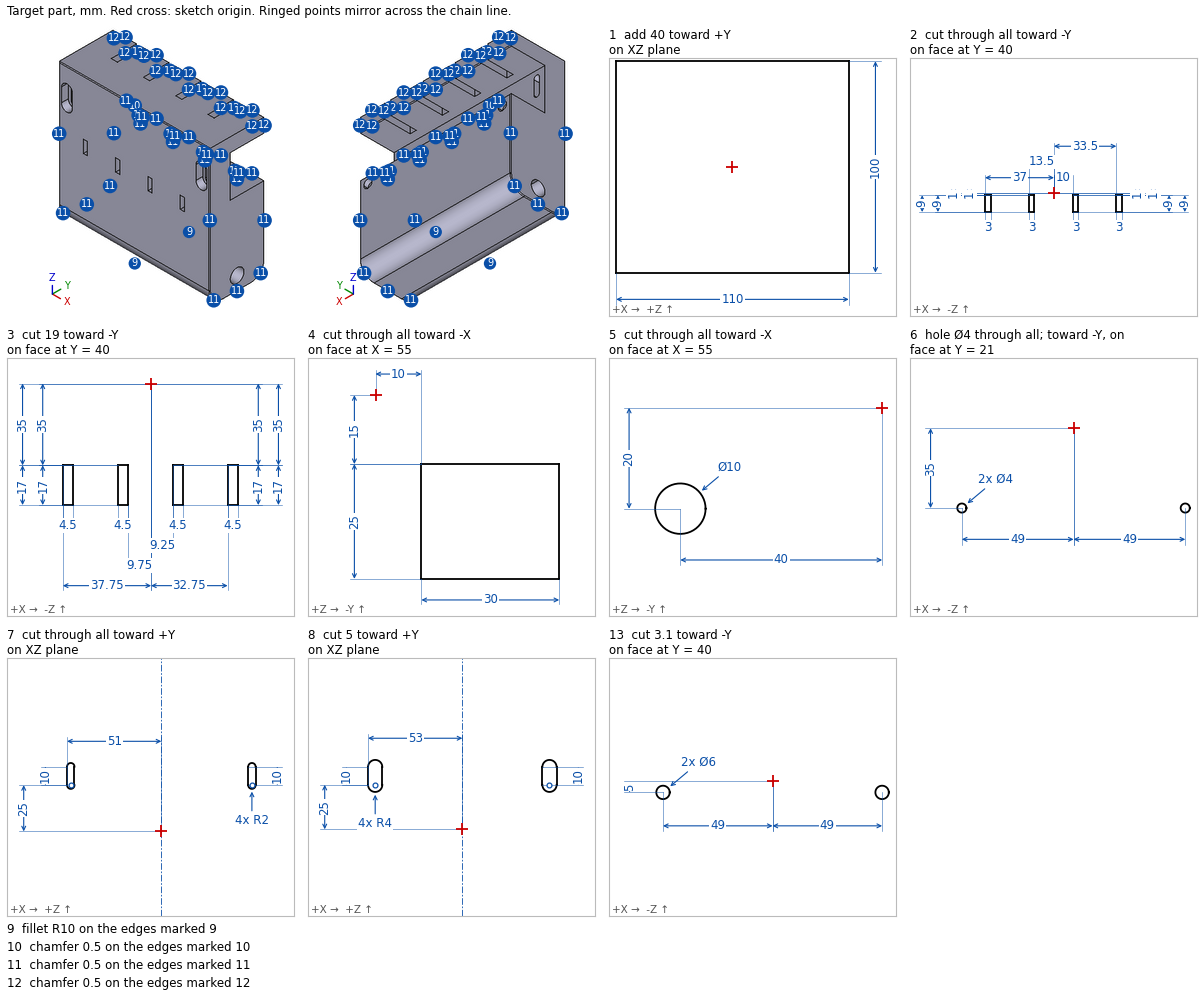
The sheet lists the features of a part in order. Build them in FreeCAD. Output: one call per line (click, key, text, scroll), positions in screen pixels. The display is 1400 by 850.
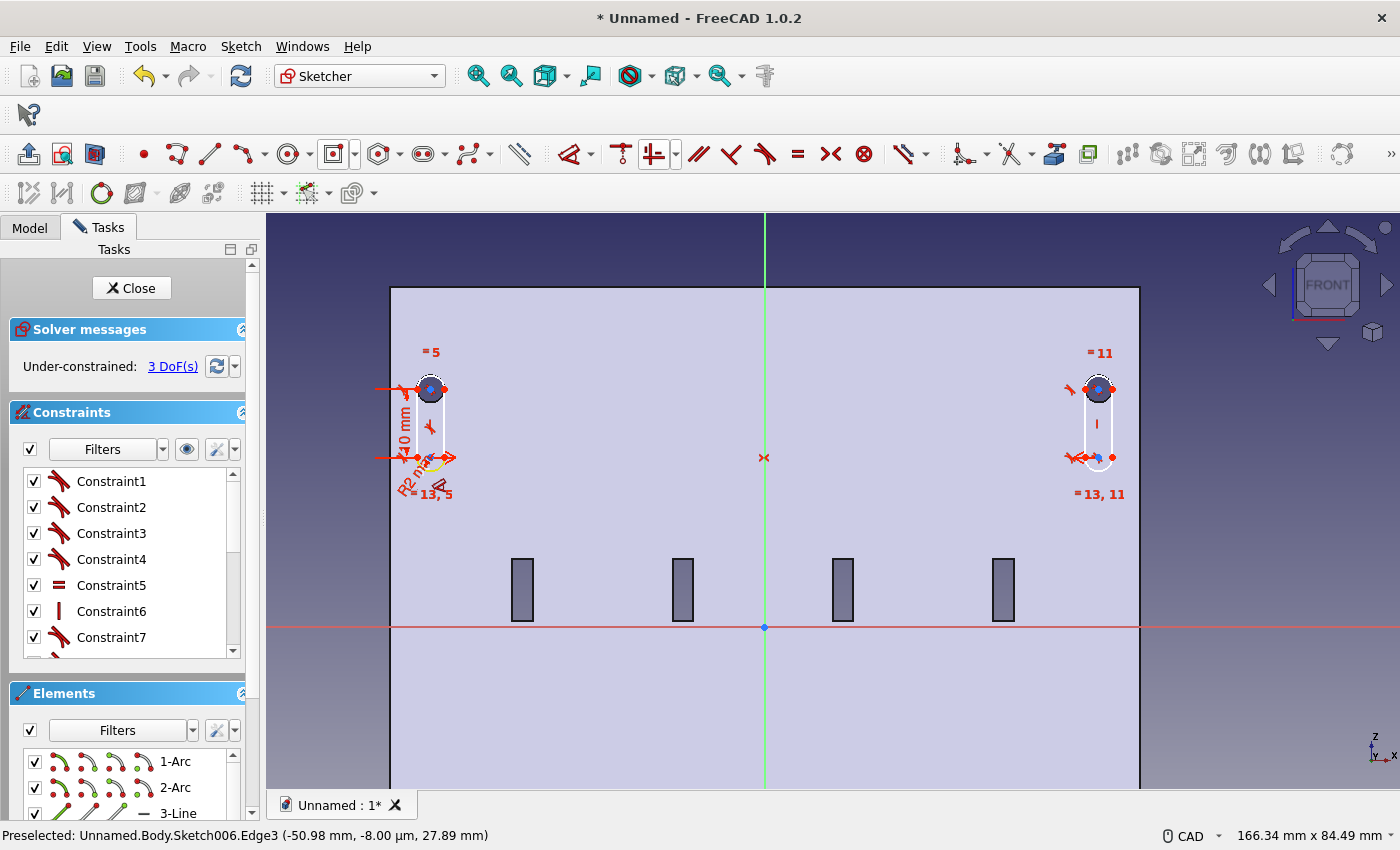
click(1085, 437)
click(1051, 424)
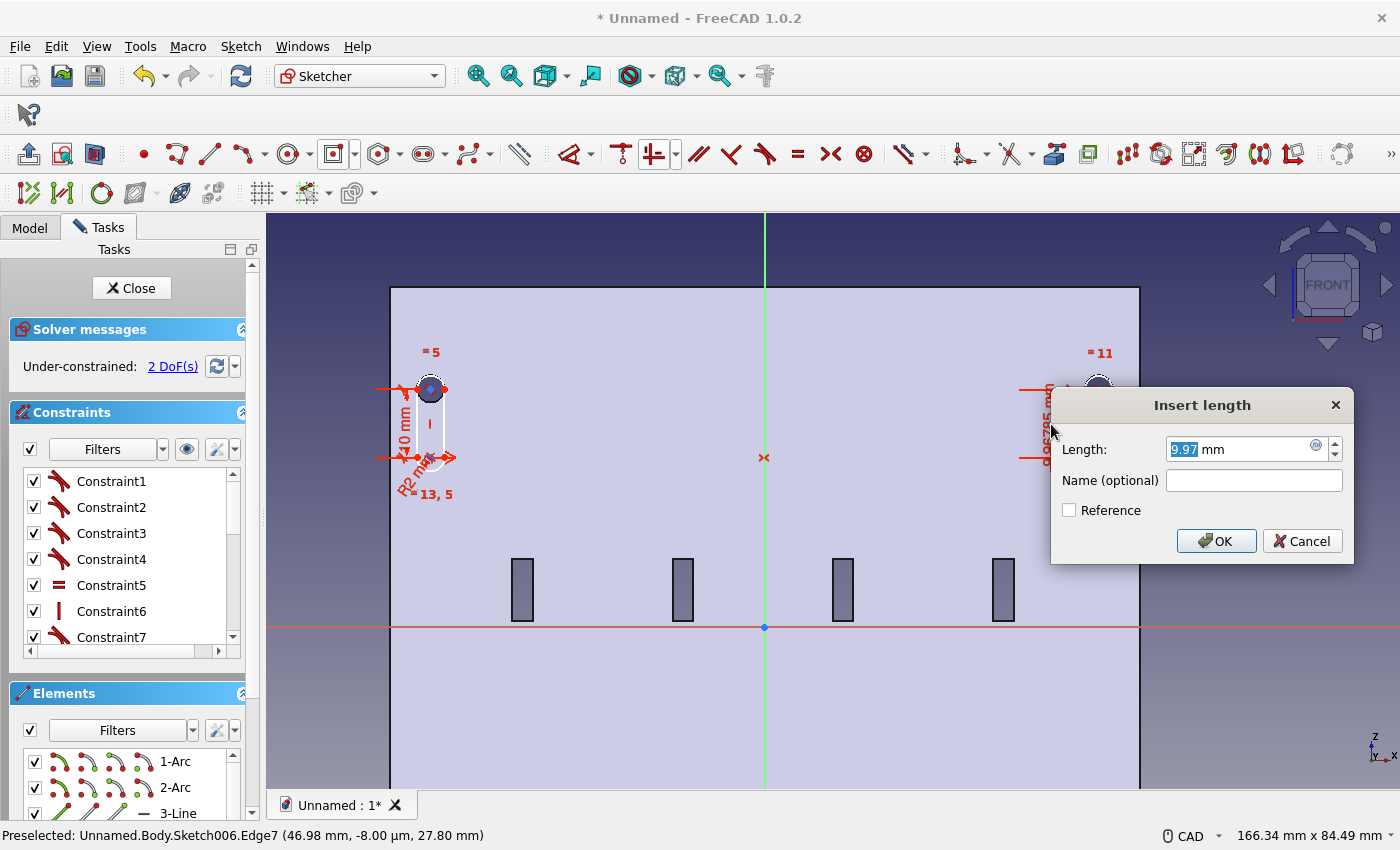
text(10)
key(Return)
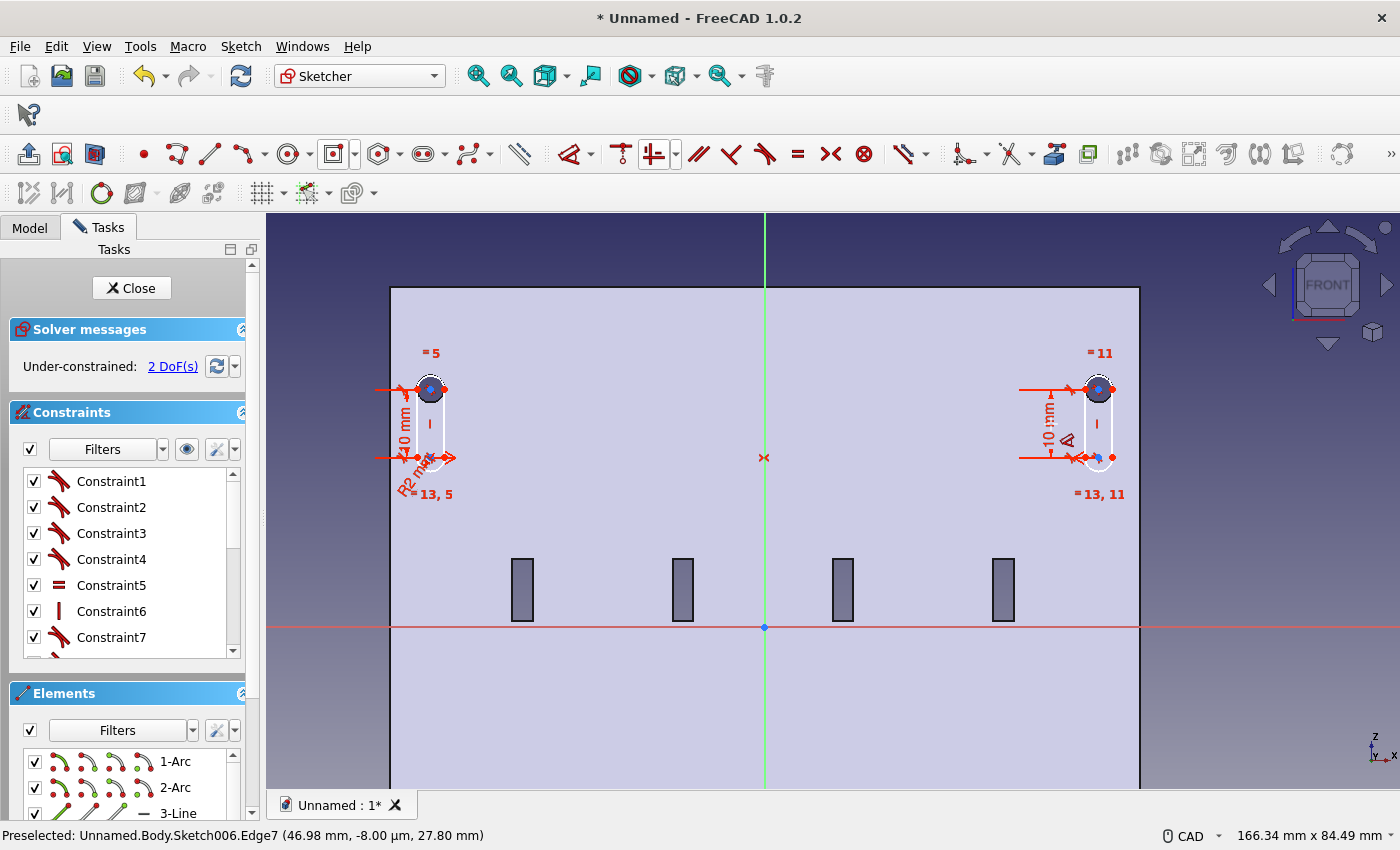
click(417, 458)
click(591, 661)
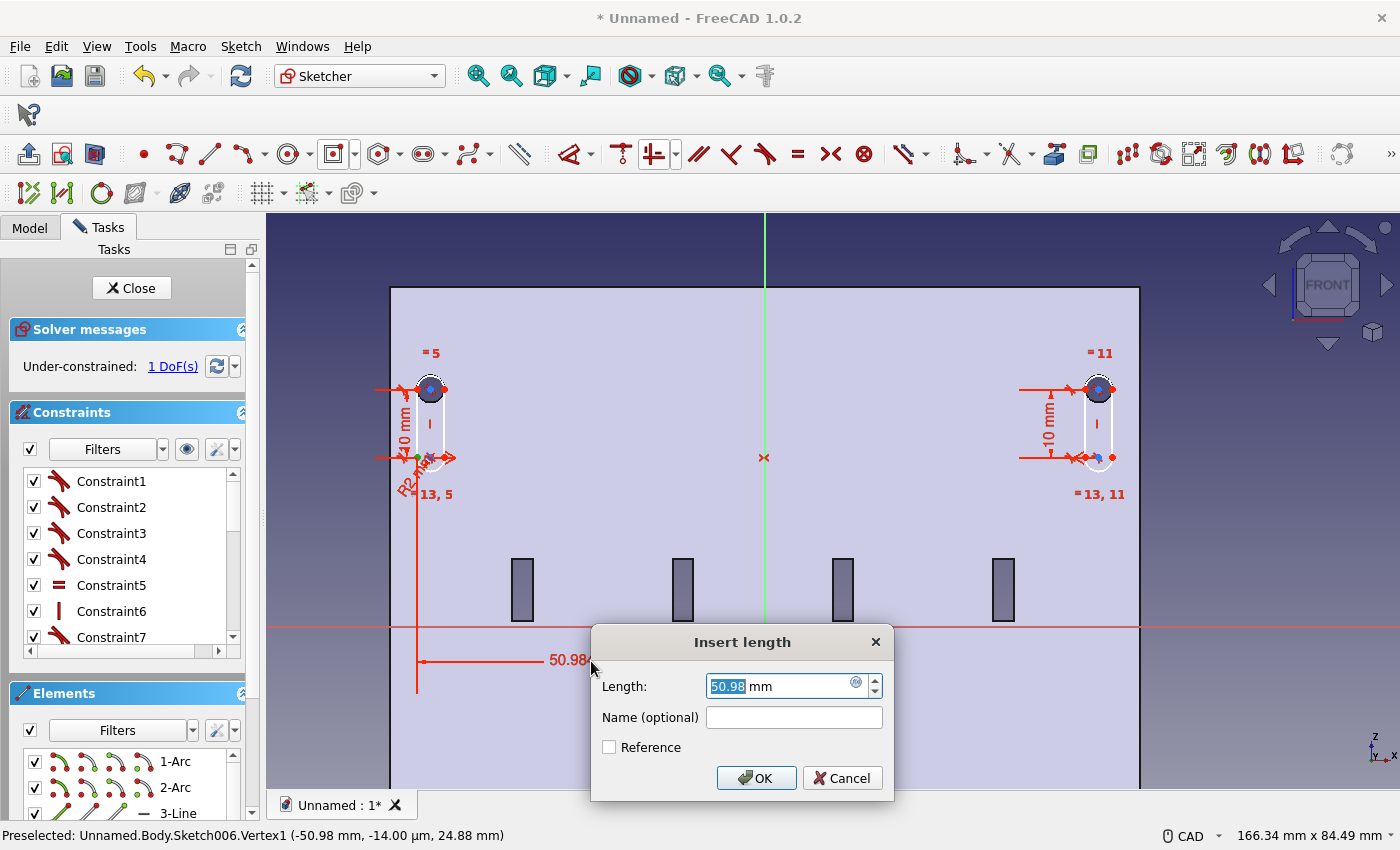
text(51)
key(Return)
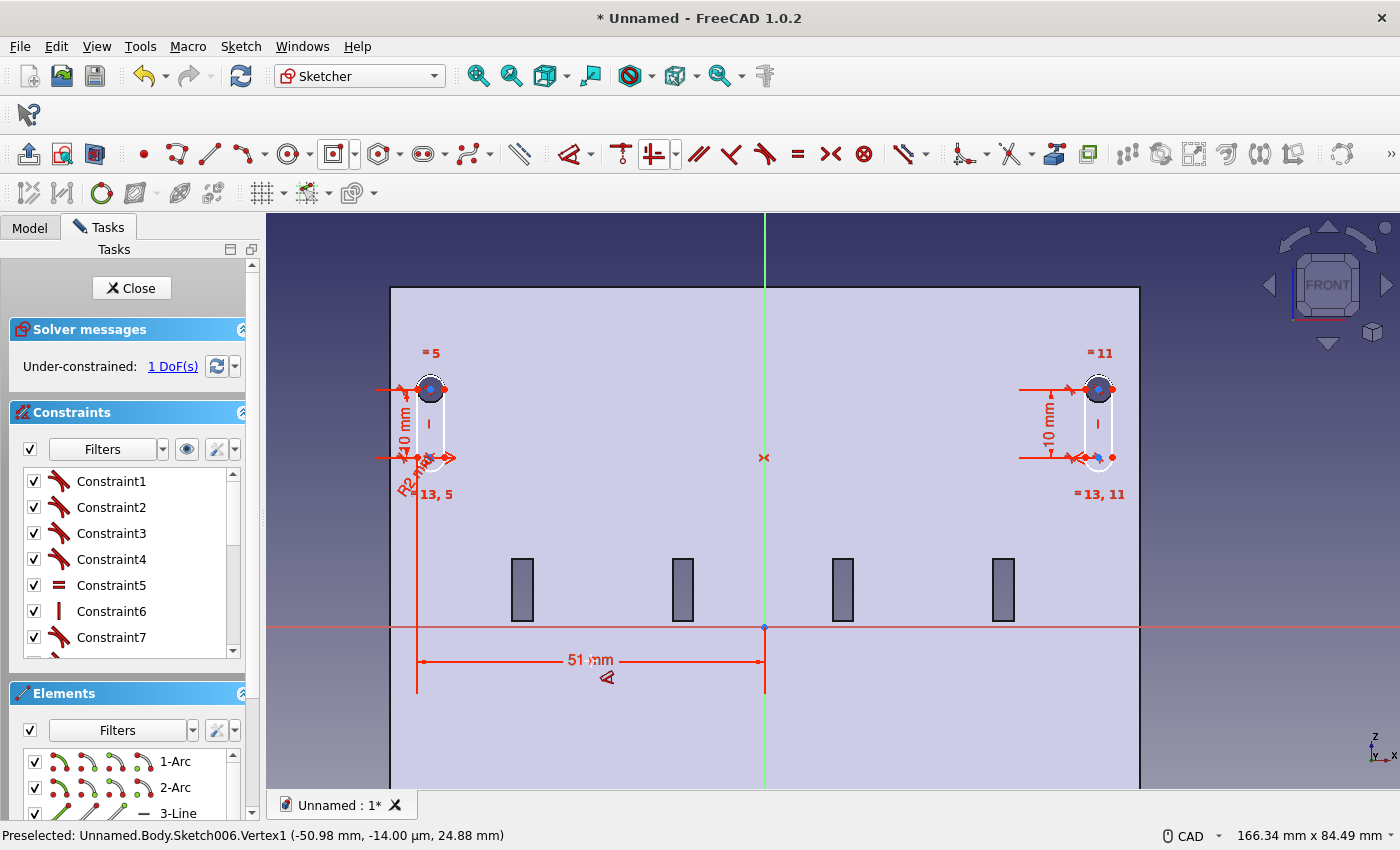
click(417, 458)
click(383, 543)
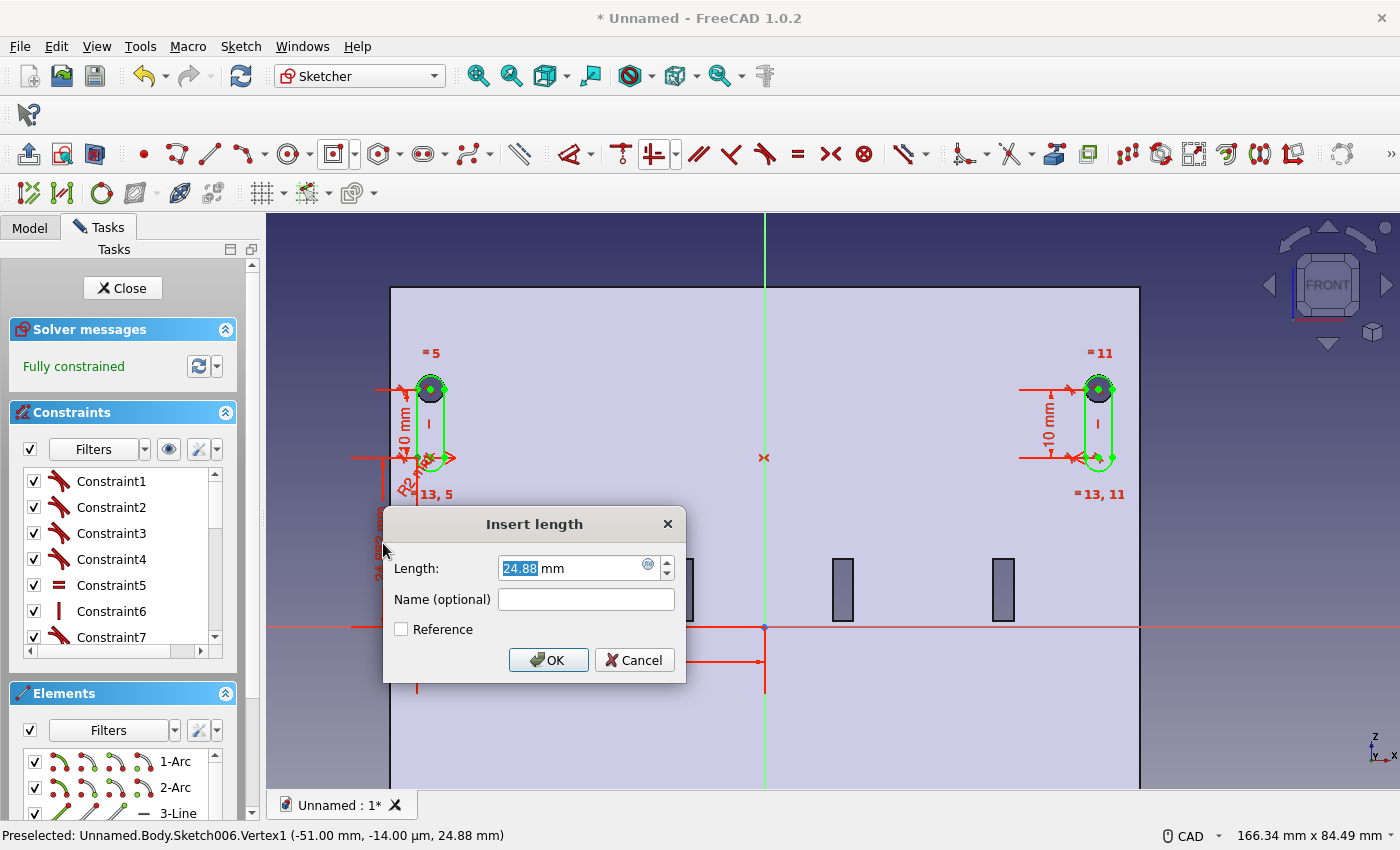
text(25)
key(Return)
key(Escape)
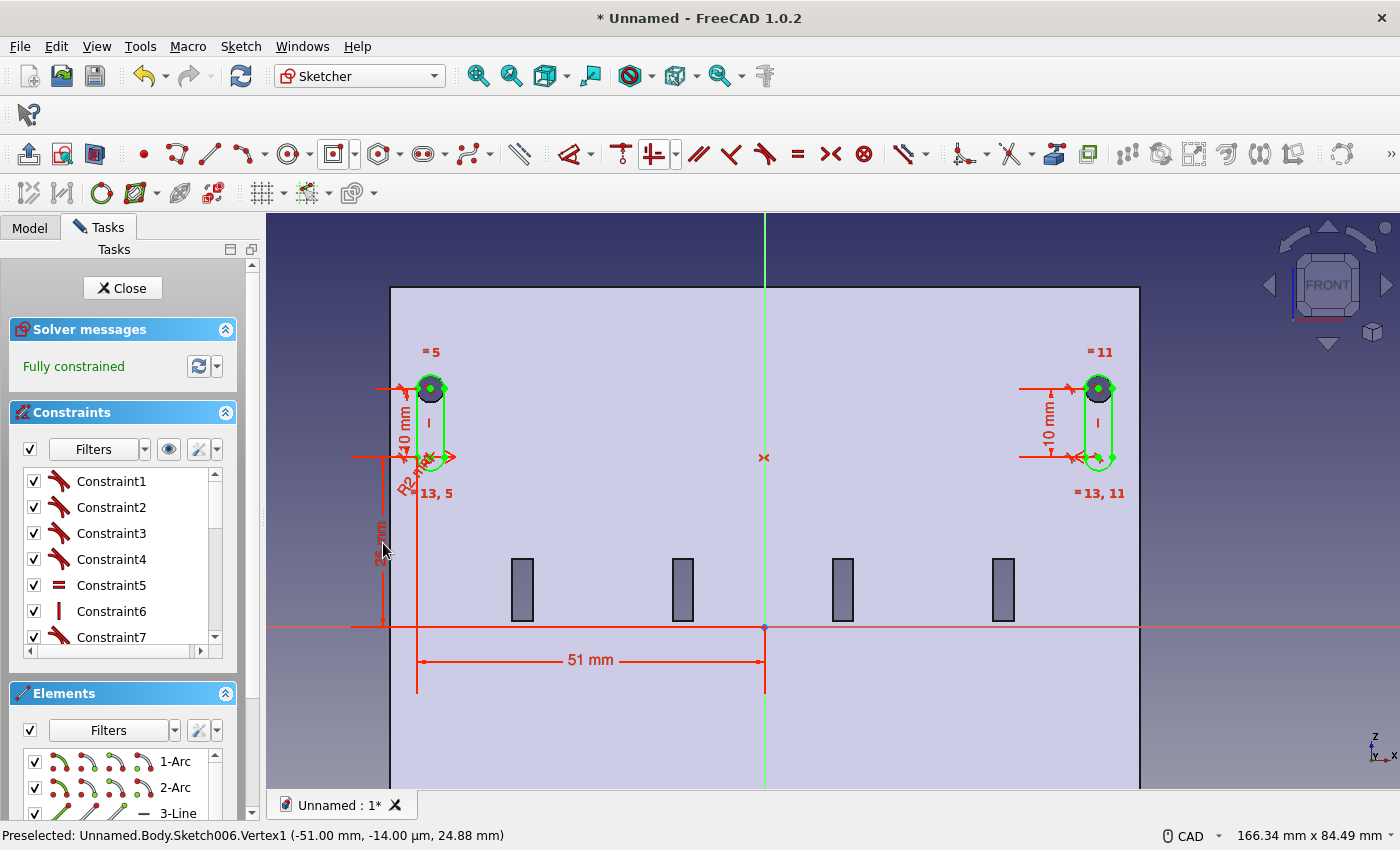
click(123, 288)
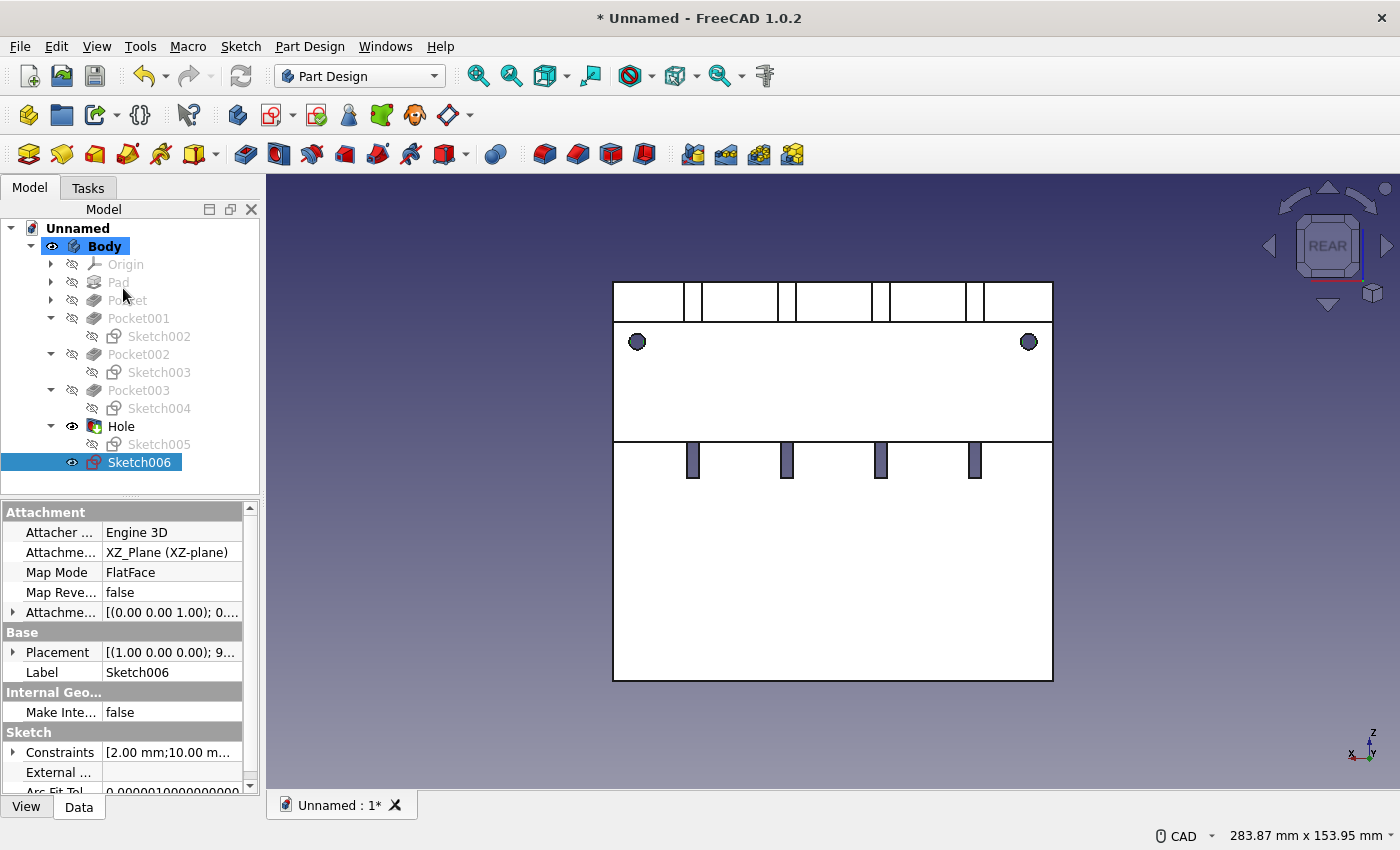
click(246, 154)